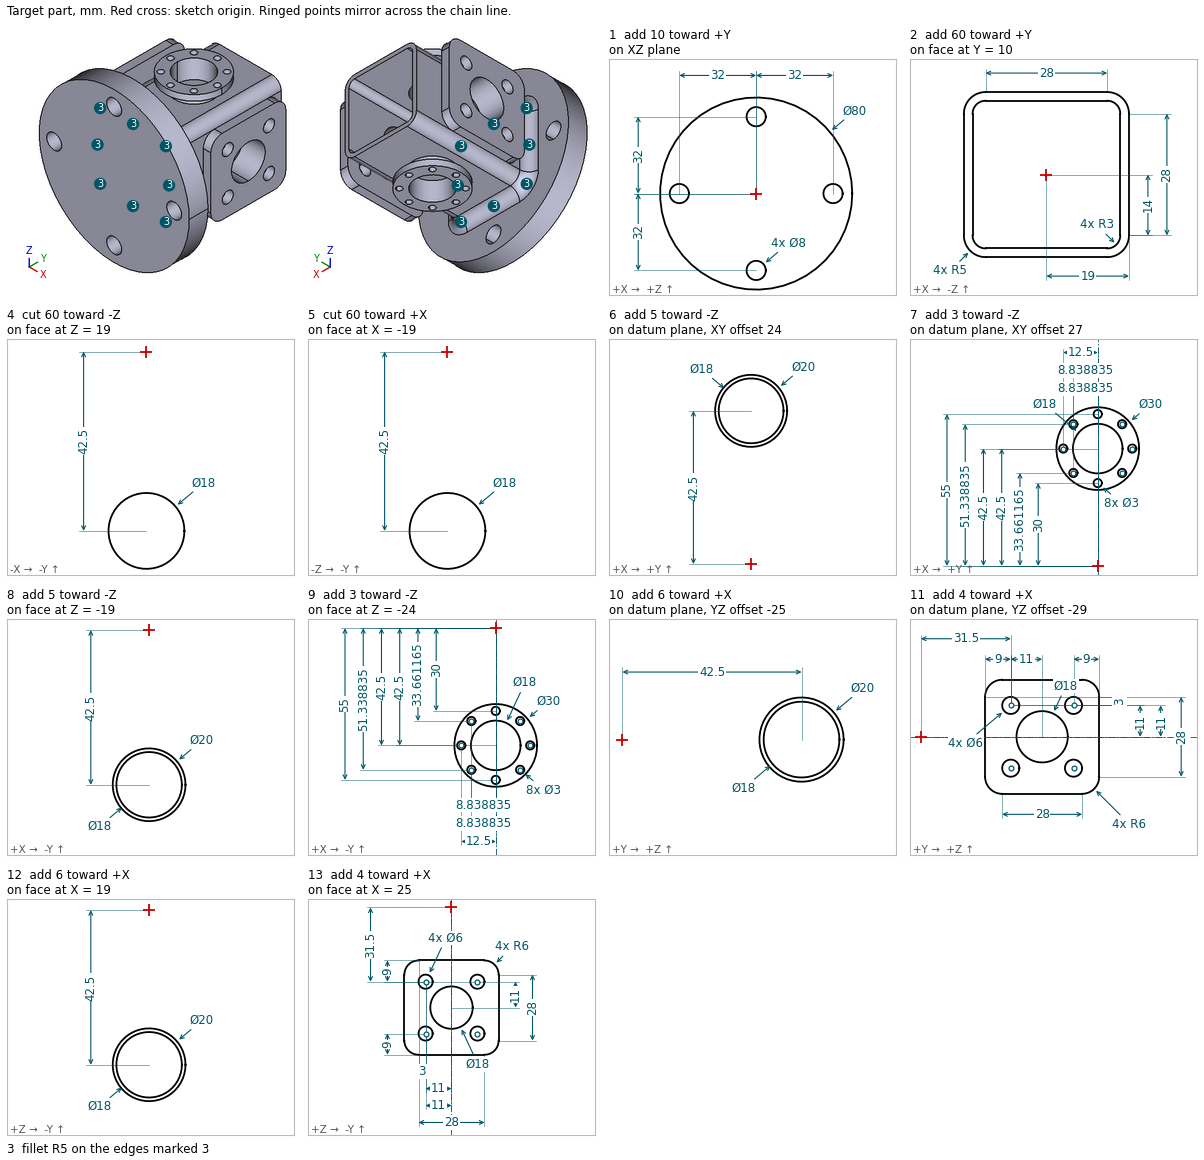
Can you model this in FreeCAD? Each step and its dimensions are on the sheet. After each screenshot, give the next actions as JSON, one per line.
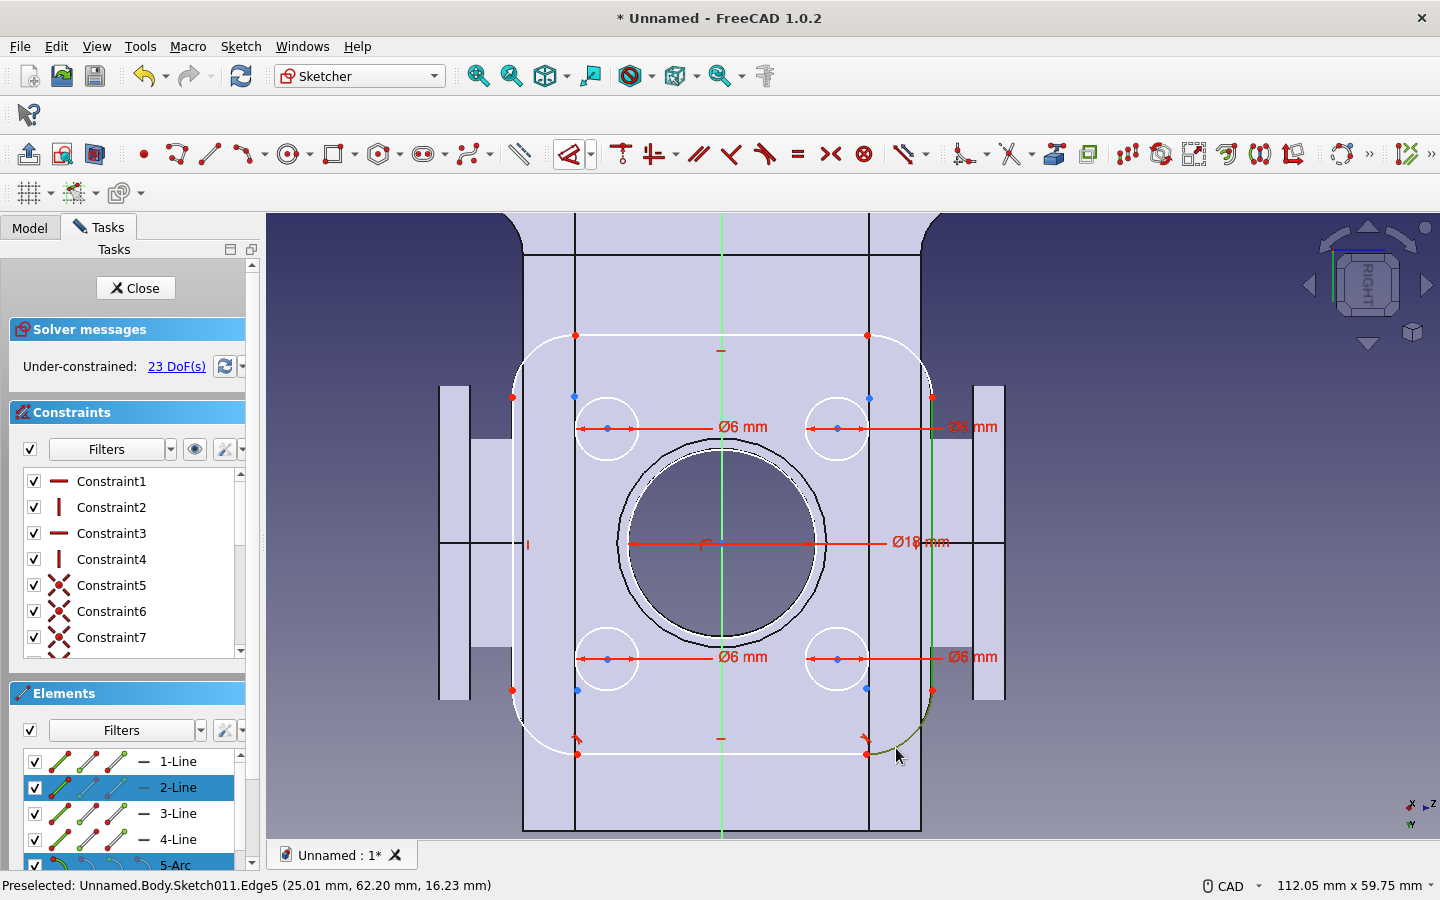
{"action": "left_click", "coordinate": [765, 154]}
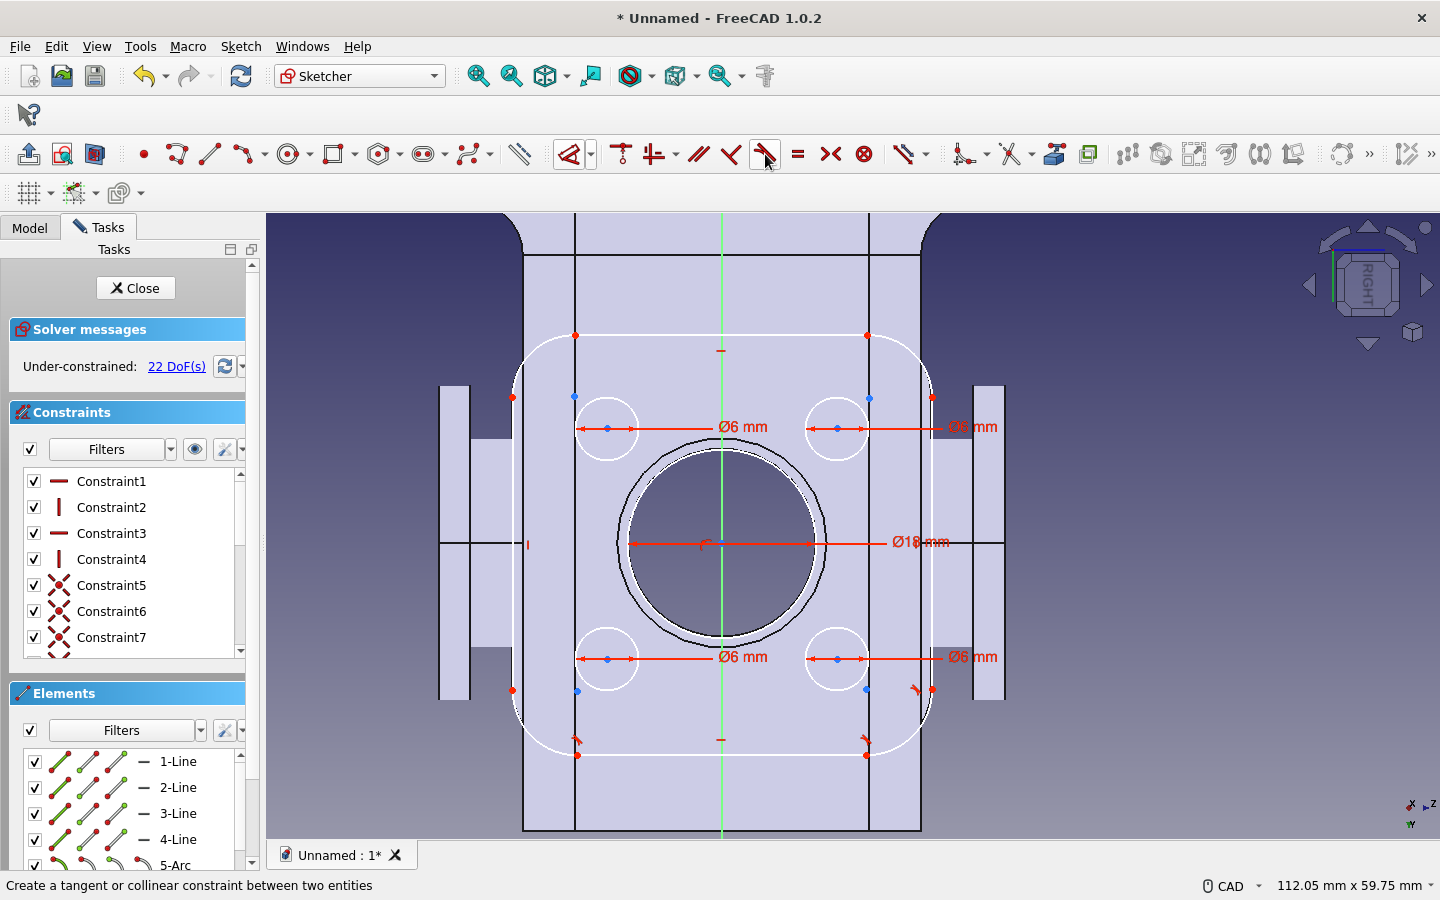
{"action": "left_click", "coordinate": [932, 602]}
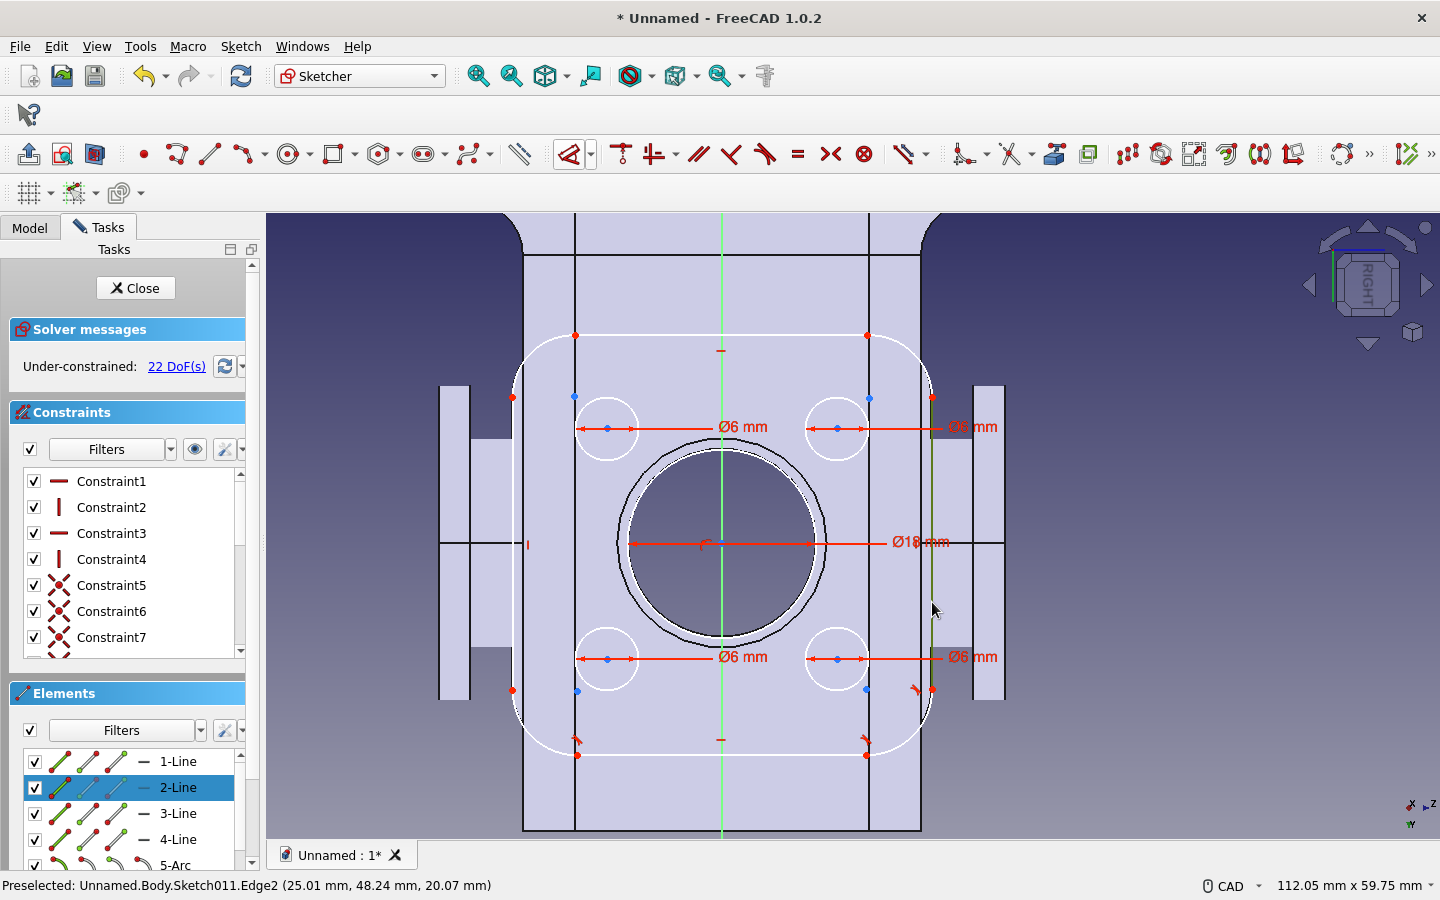
{"action": "left_click", "coordinate": [925, 369]}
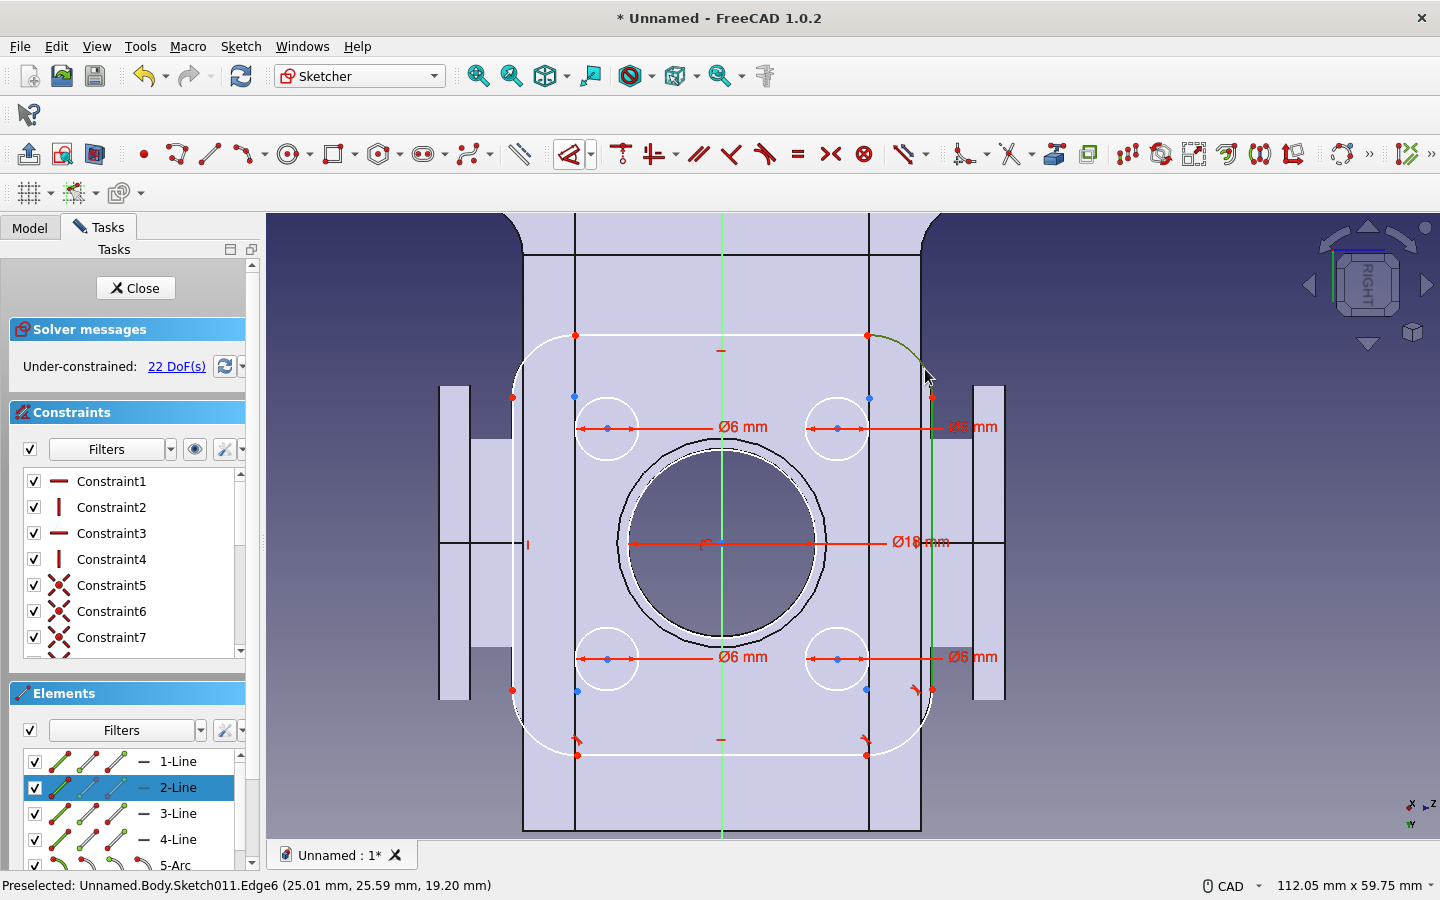
{"action": "left_click", "coordinate": [765, 154]}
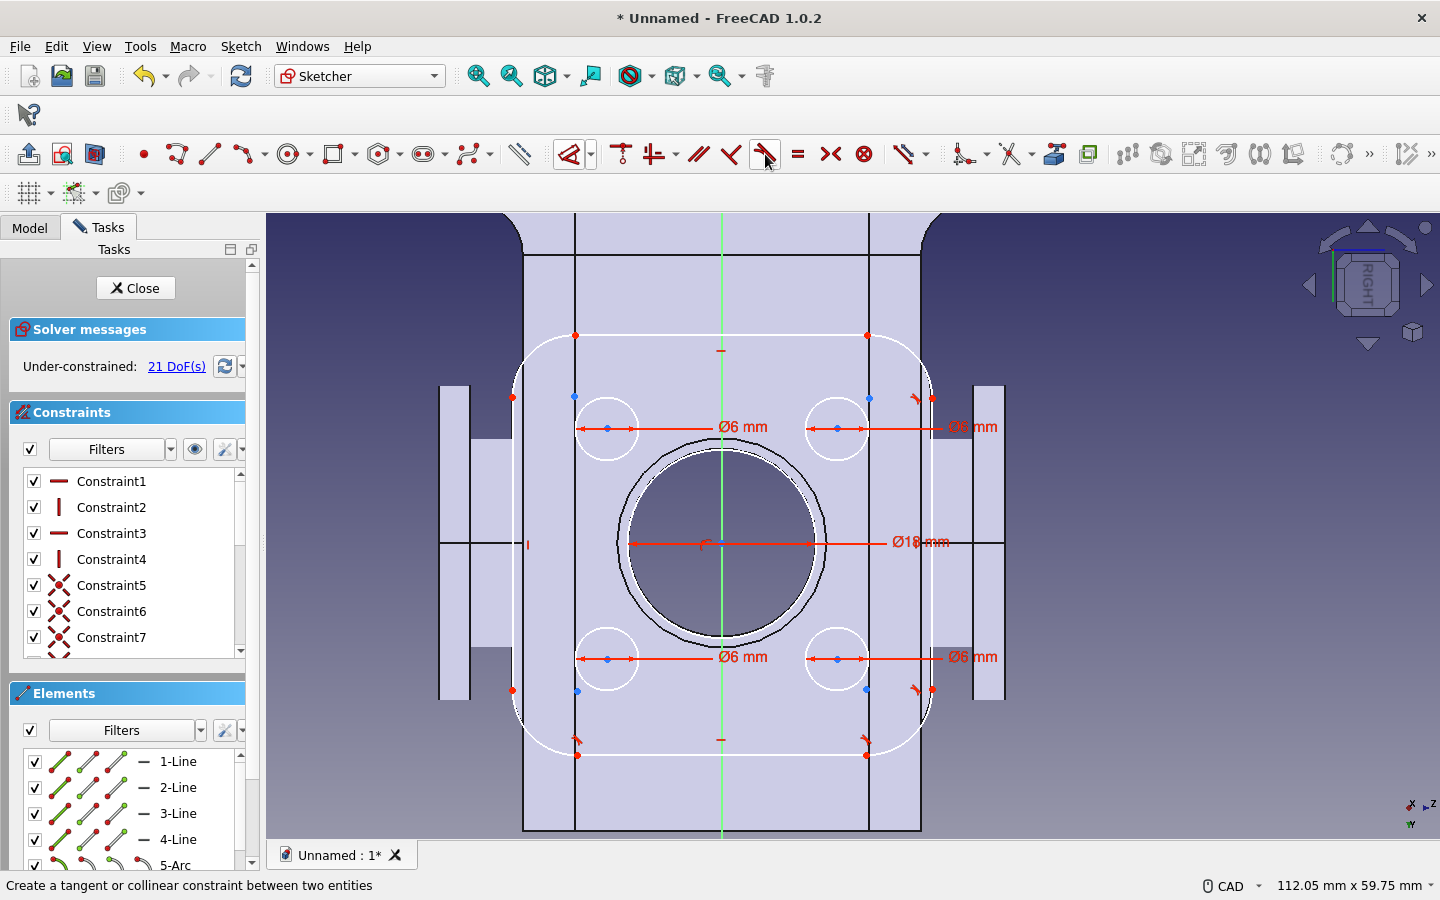
{"action": "left_click", "coordinate": [780, 335]}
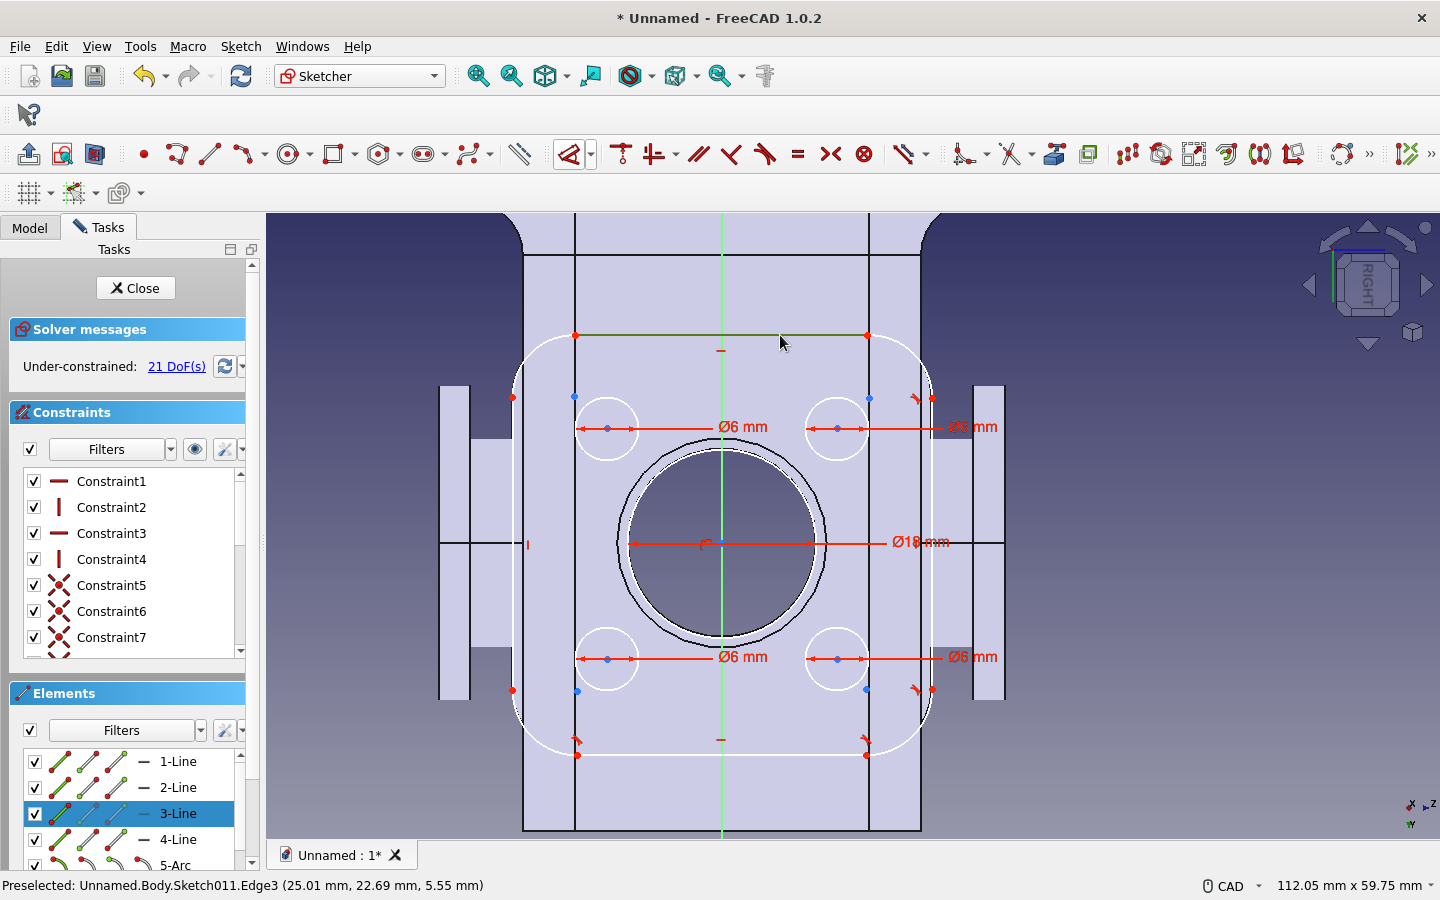
{"action": "left_click", "coordinate": [925, 369]}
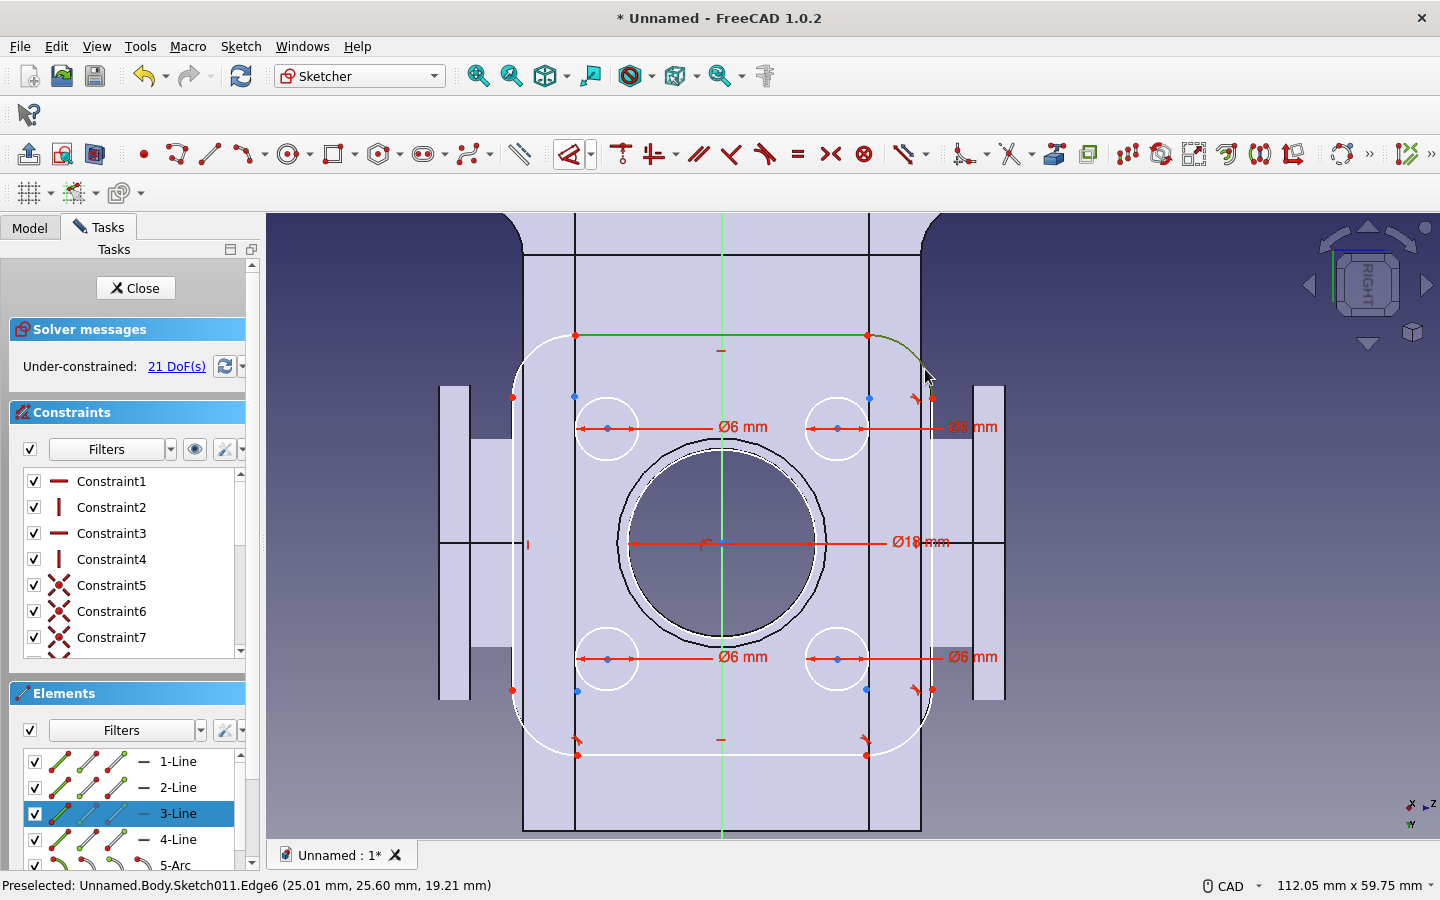
{"action": "key", "text": "t"}